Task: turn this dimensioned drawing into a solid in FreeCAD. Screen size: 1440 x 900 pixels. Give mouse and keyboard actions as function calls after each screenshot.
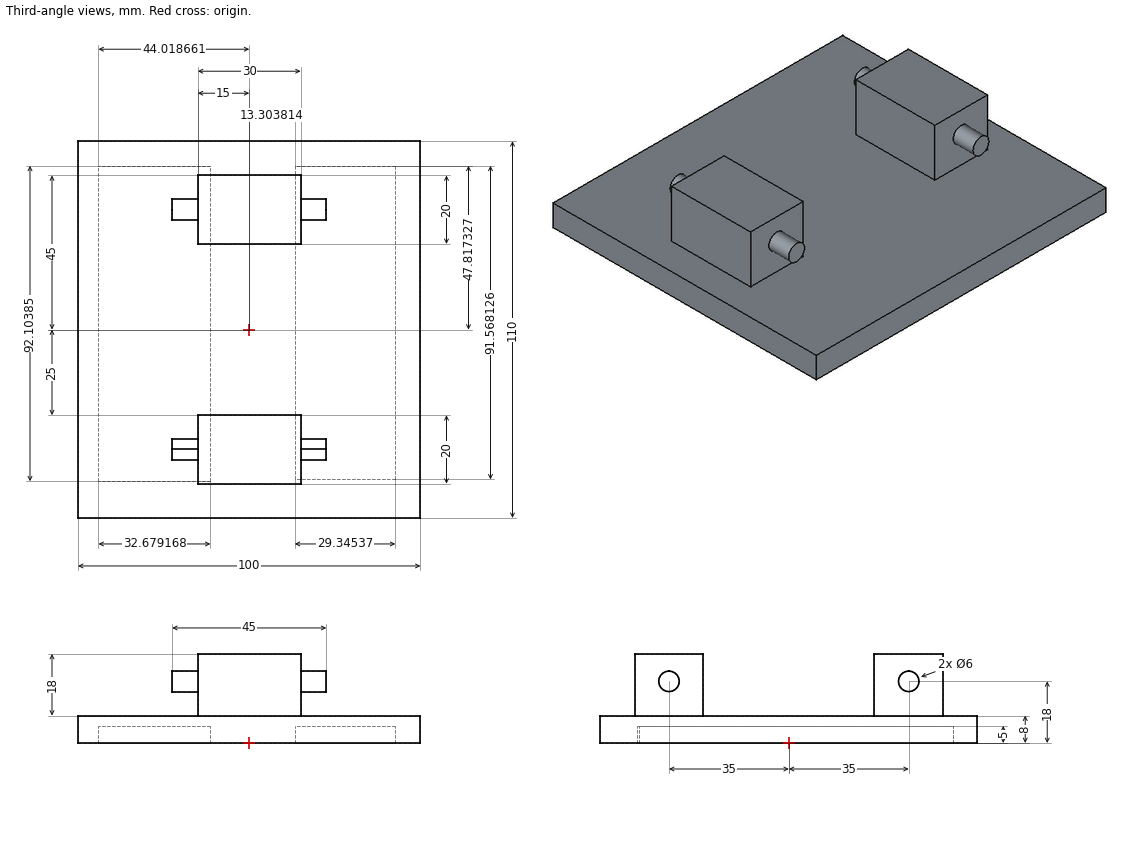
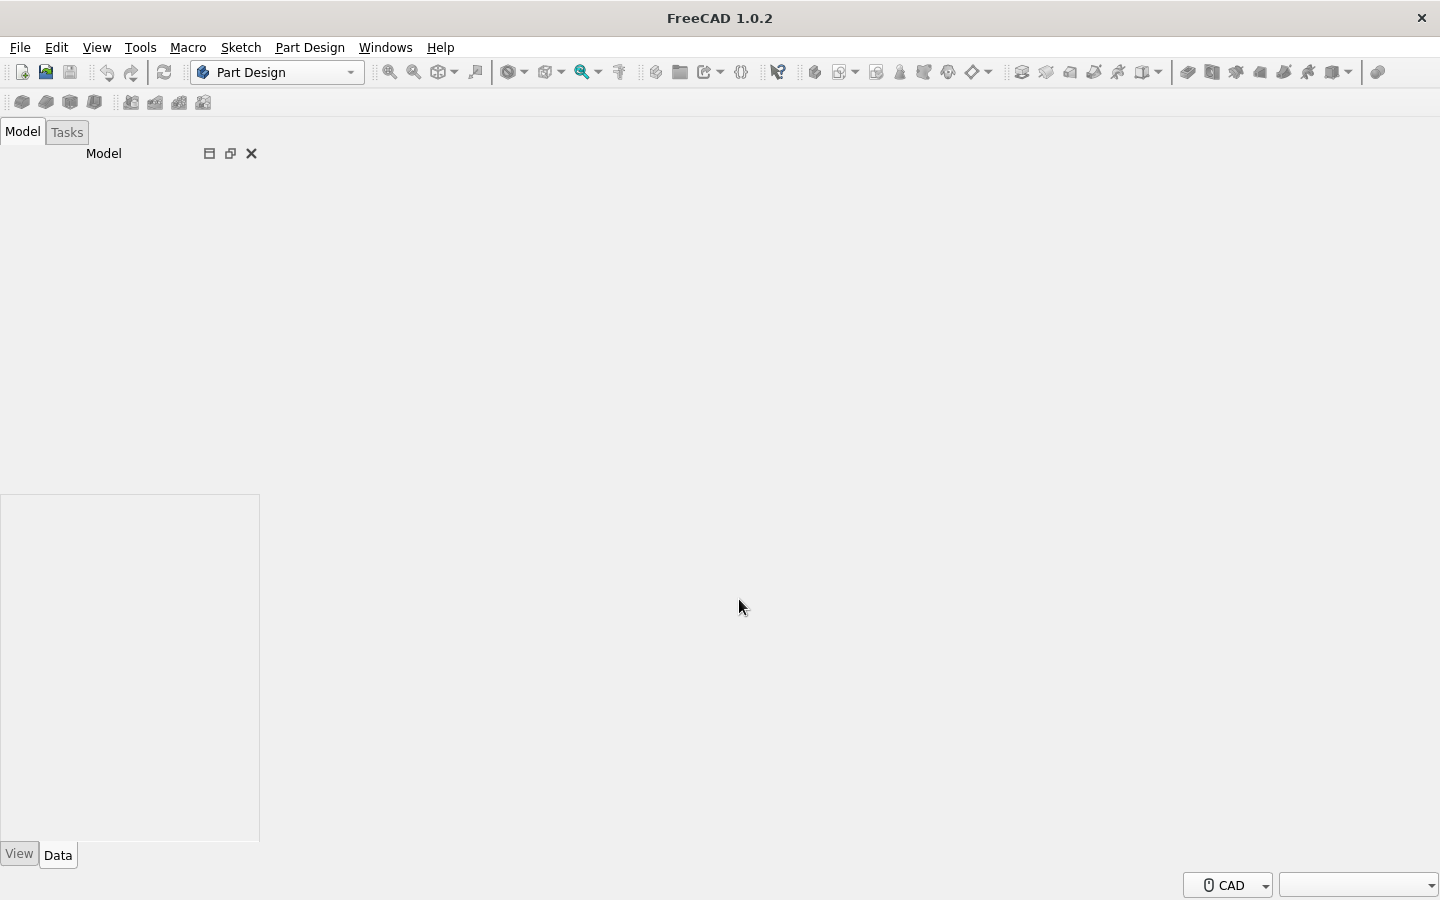
key(ctrl+n)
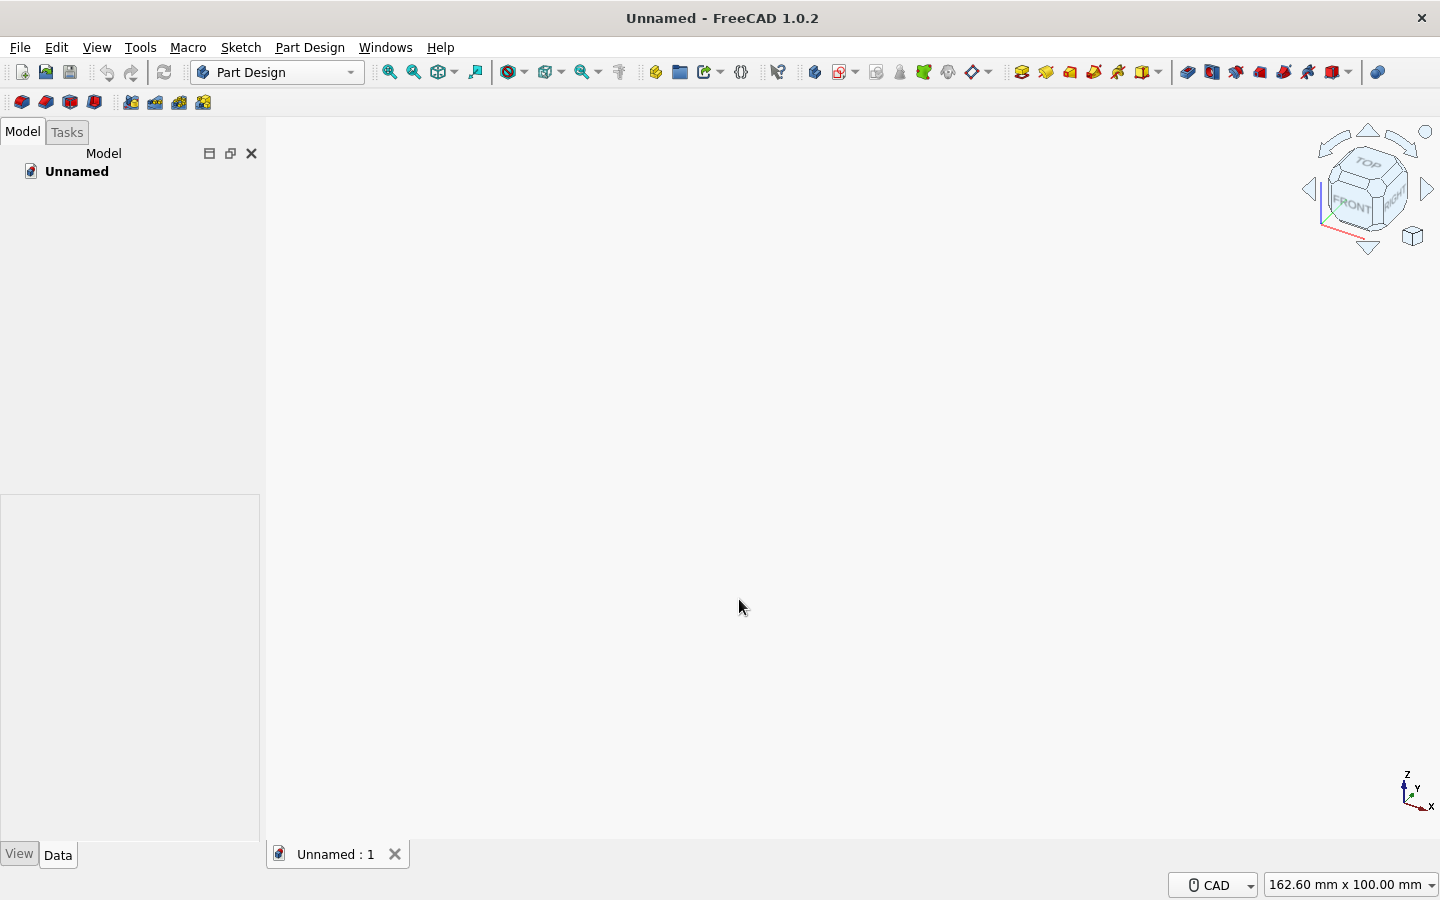
click(840, 72)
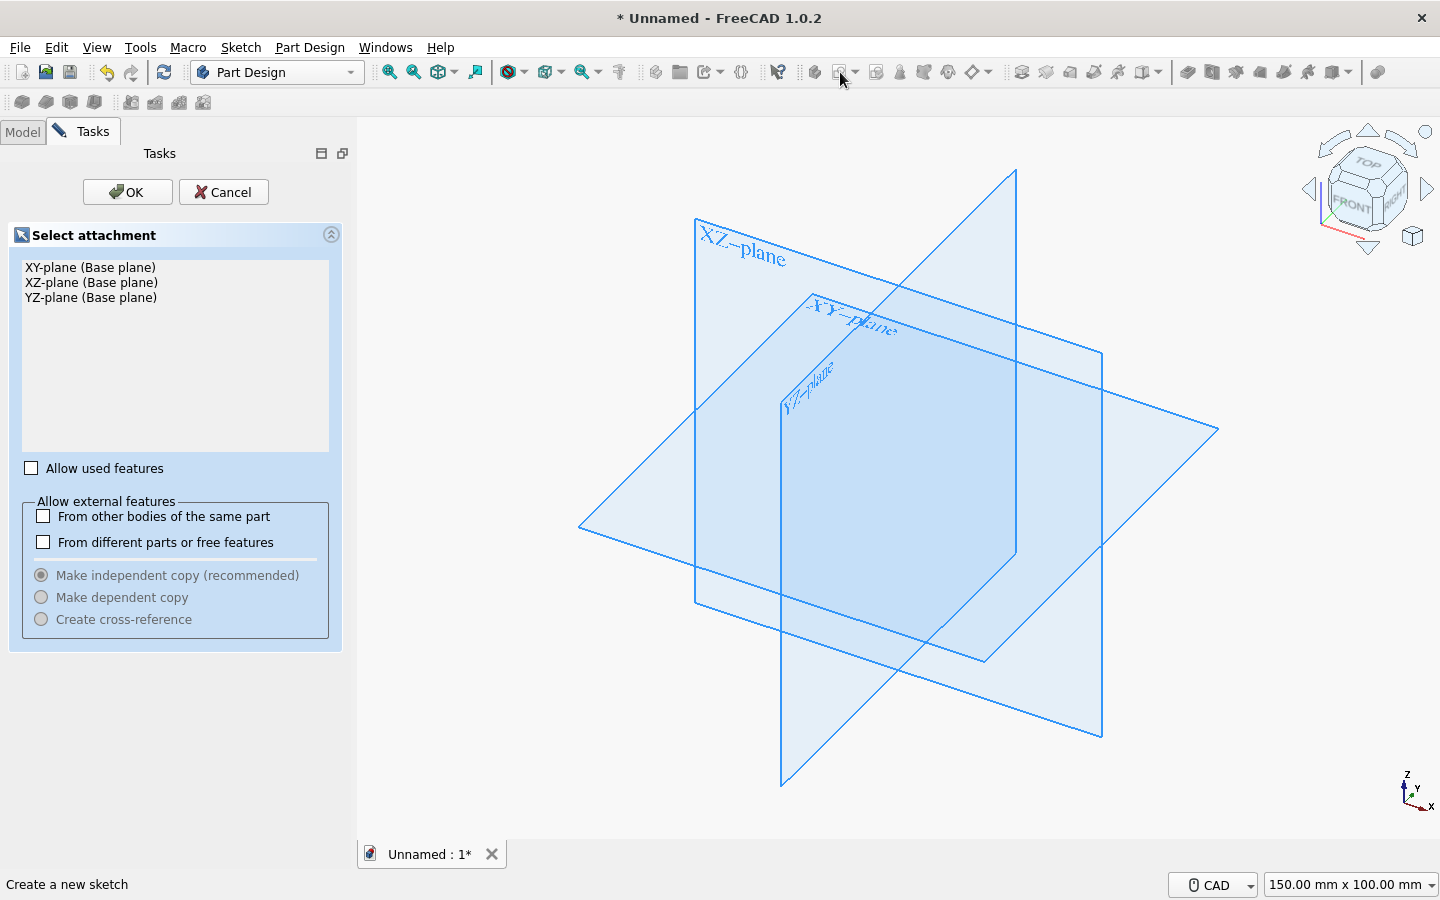
click(82, 268)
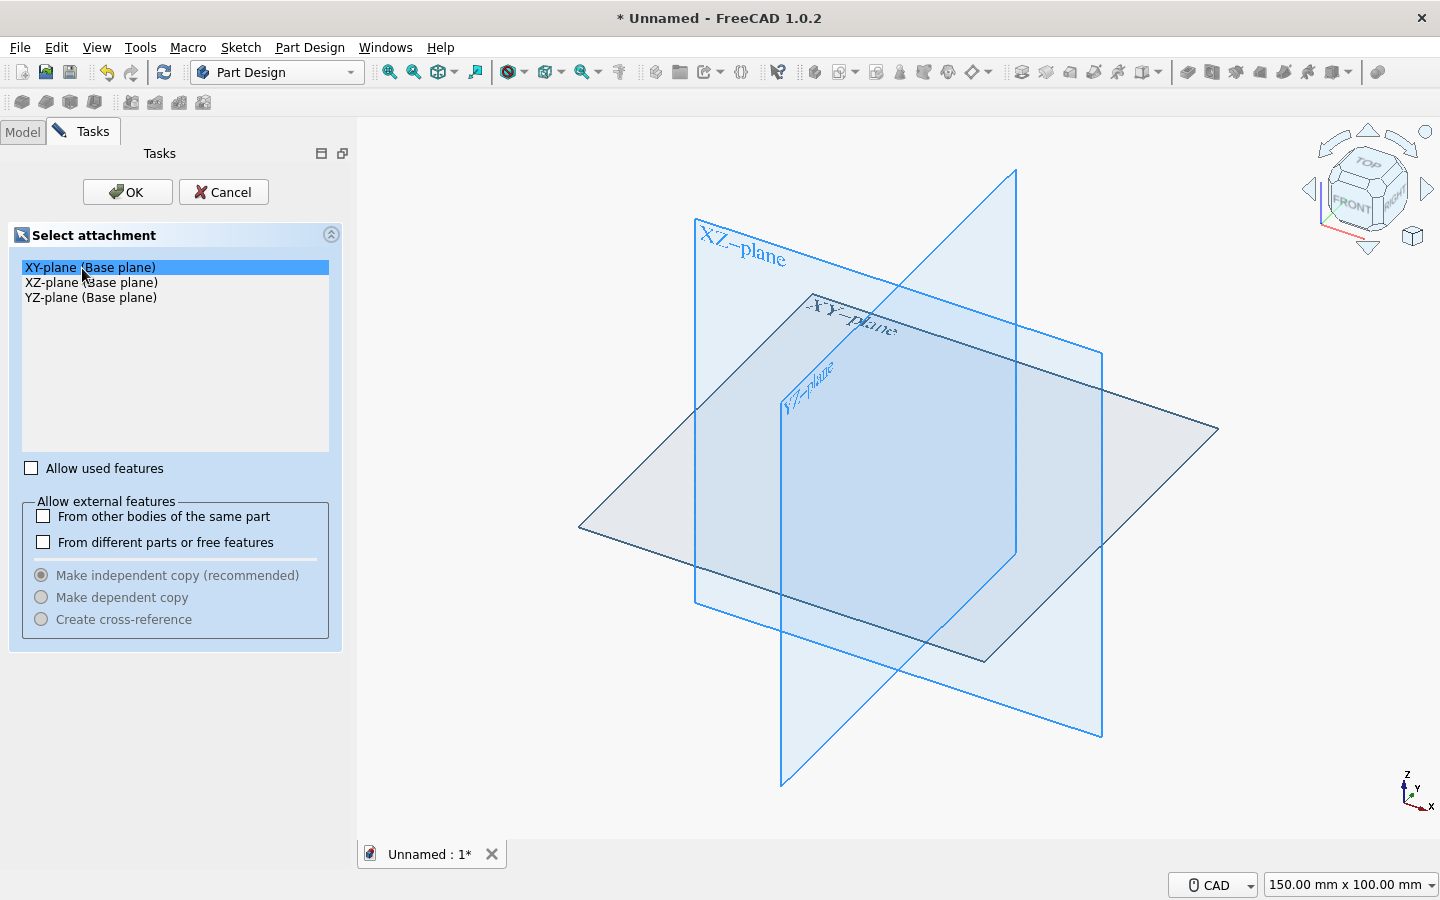
click(128, 192)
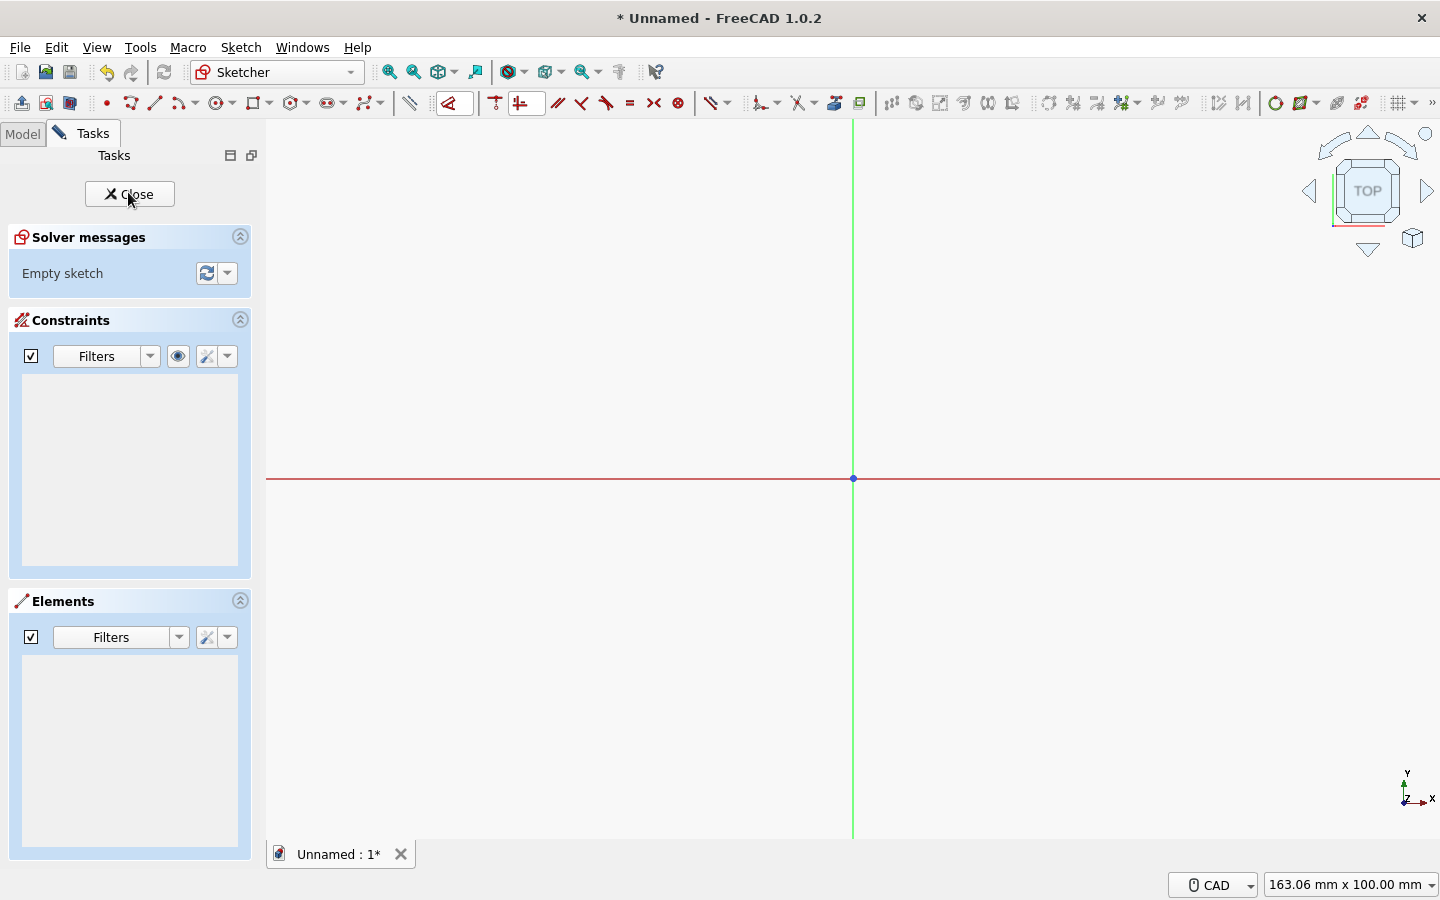
scroll(701, 479, down, 3)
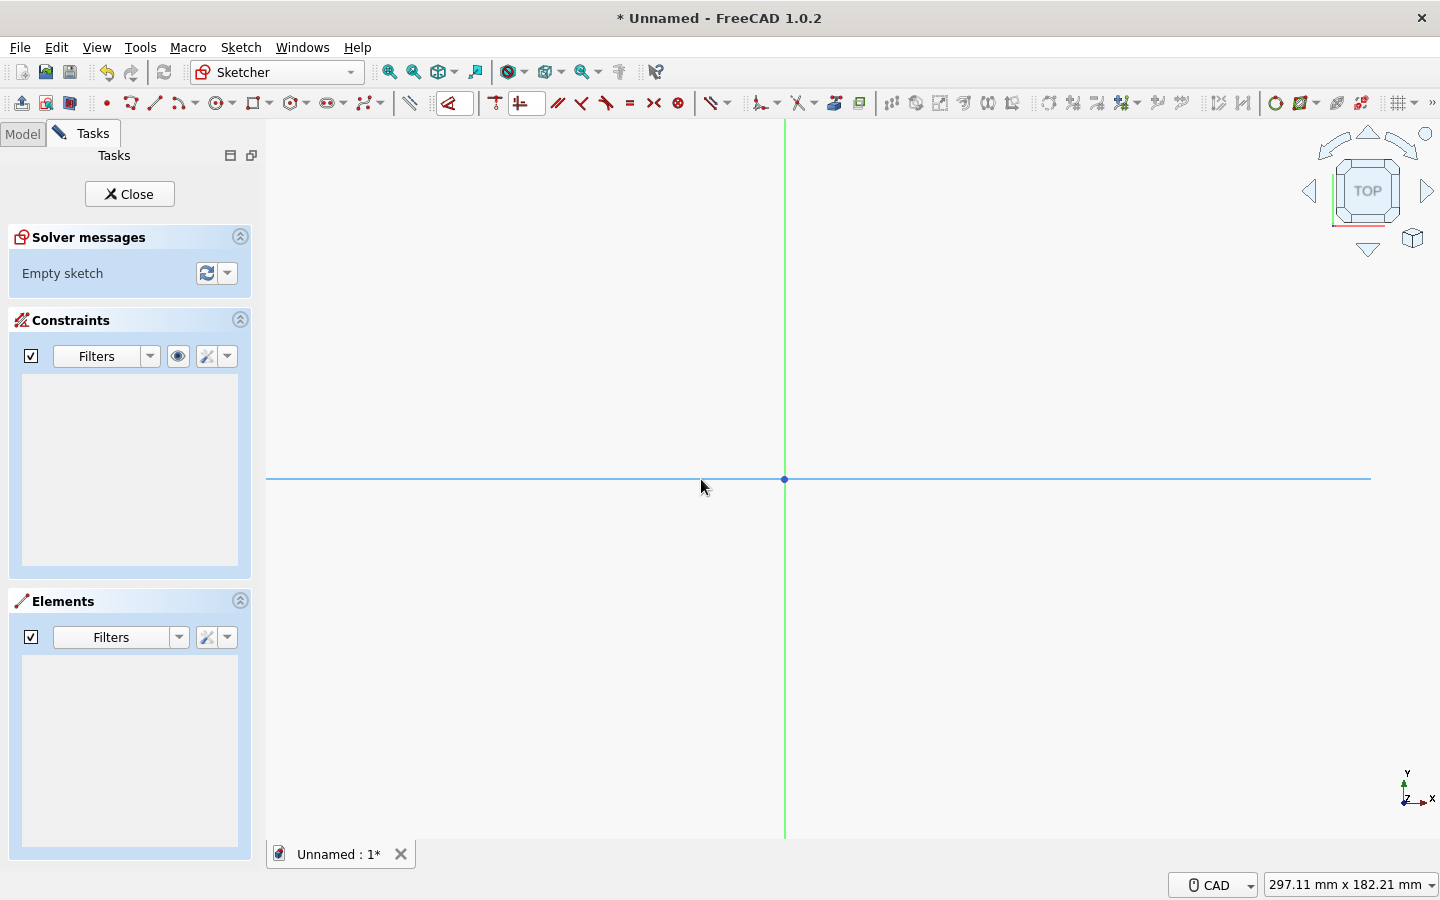
key(g)
key(v)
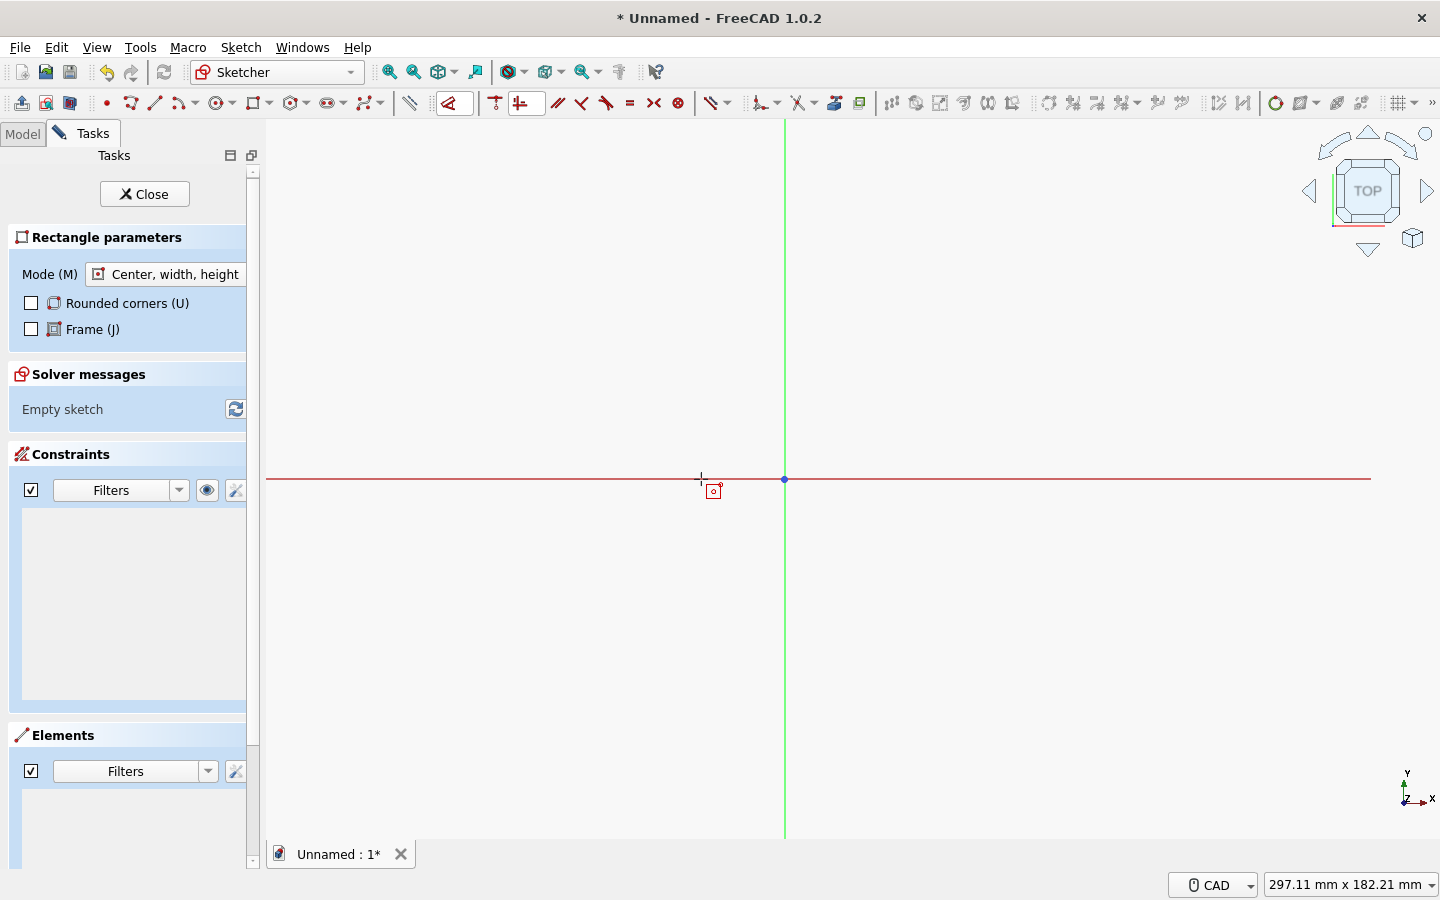
click(785, 479)
move(982, 262)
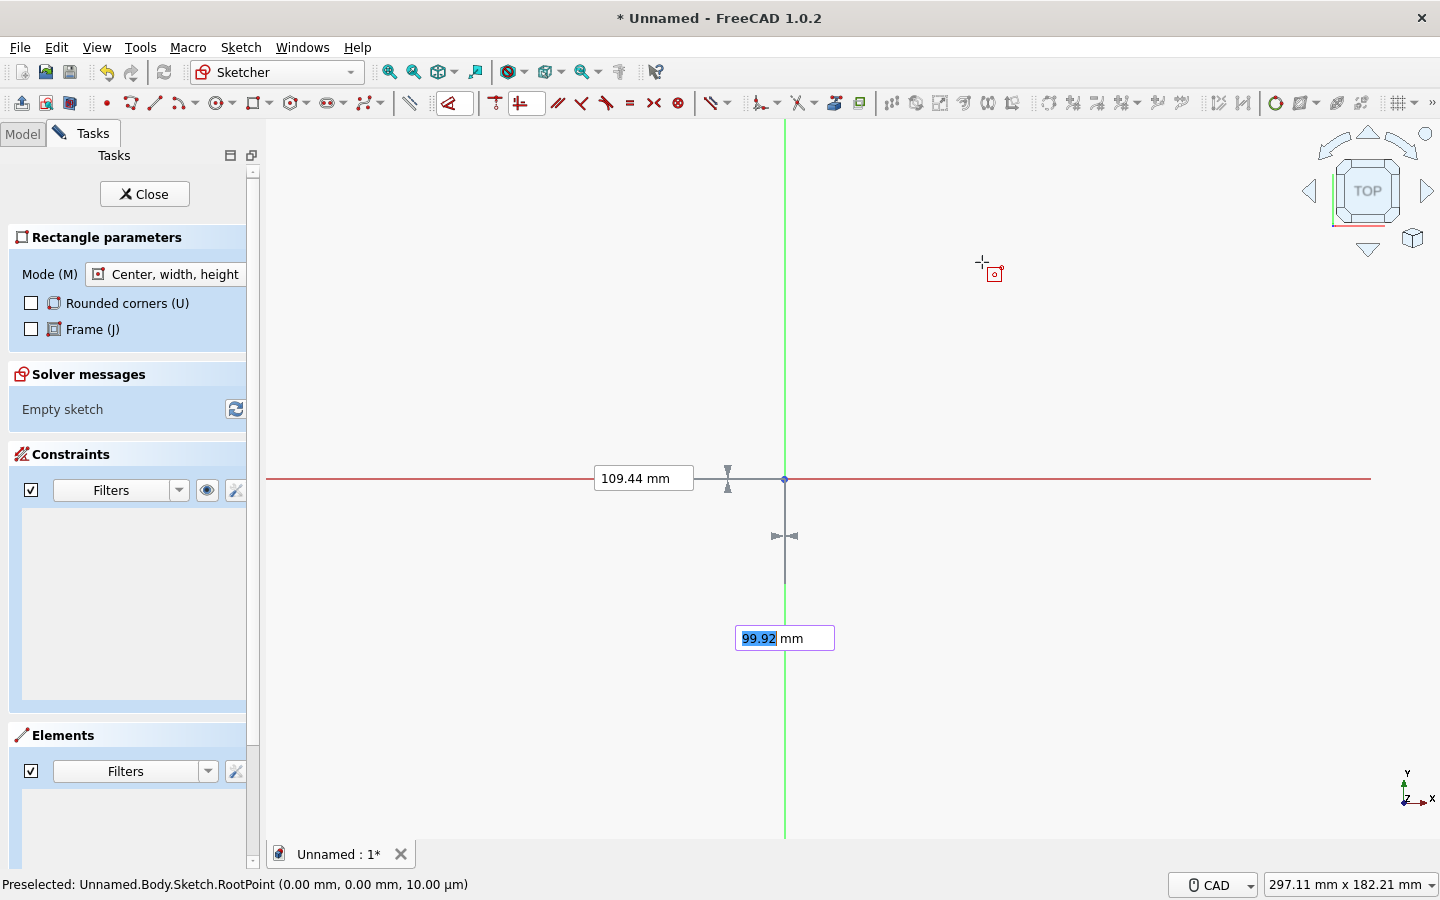
text(100)
key(Tab)
text(110)
key(Return)
key(Escape)